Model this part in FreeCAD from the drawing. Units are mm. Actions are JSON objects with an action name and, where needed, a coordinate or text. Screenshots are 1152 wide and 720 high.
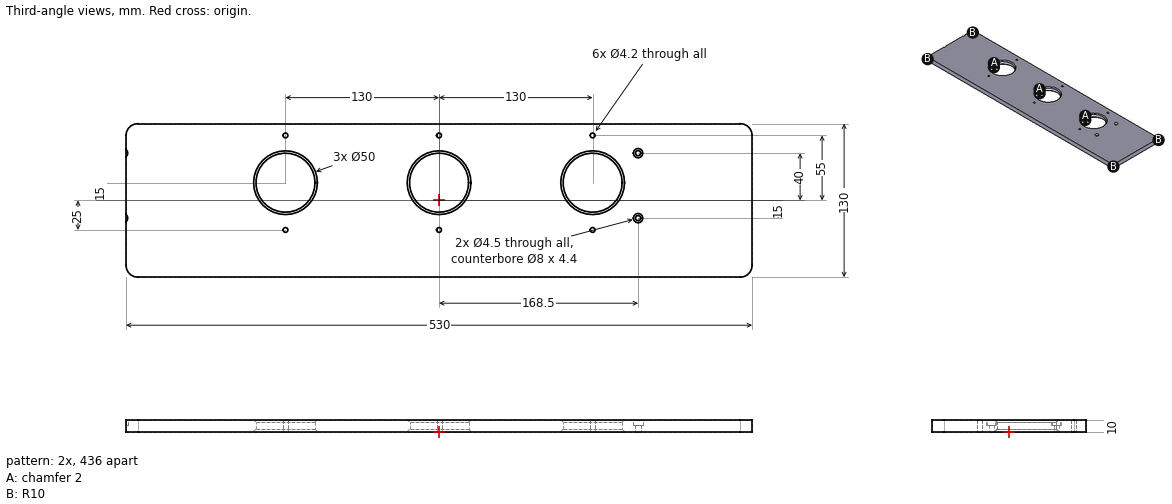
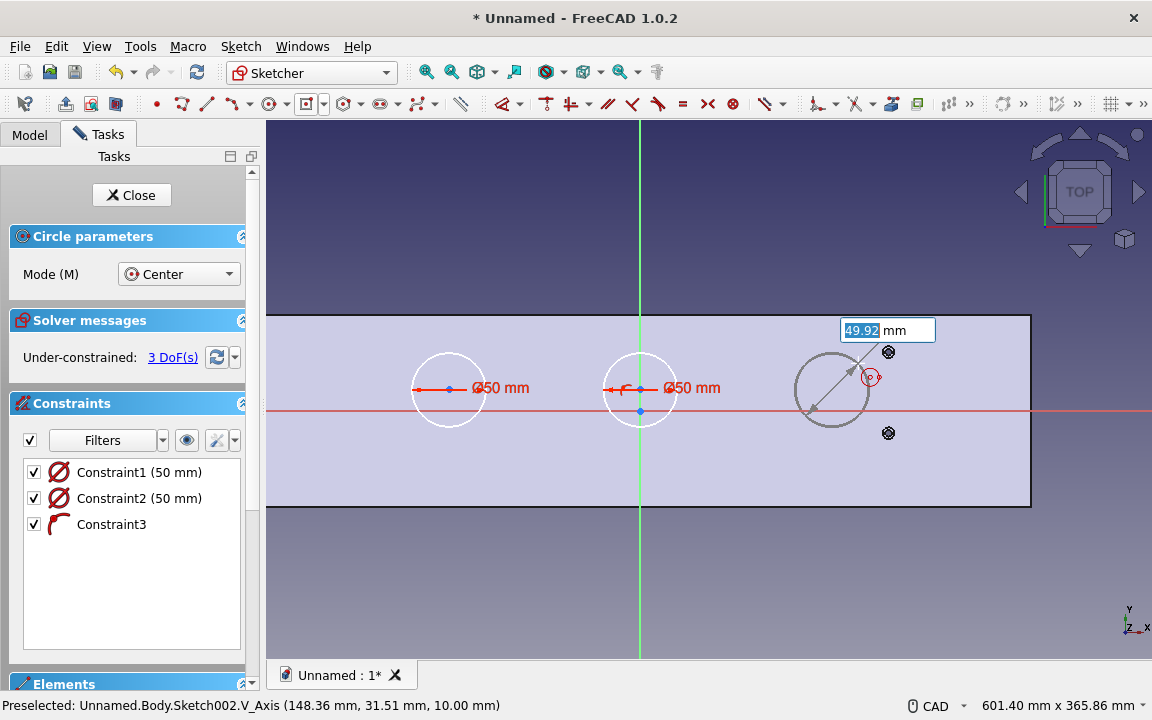
{"action": "type", "text": "50"}
{"action": "key", "text": "Return"}
{"action": "key", "text": "Escape"}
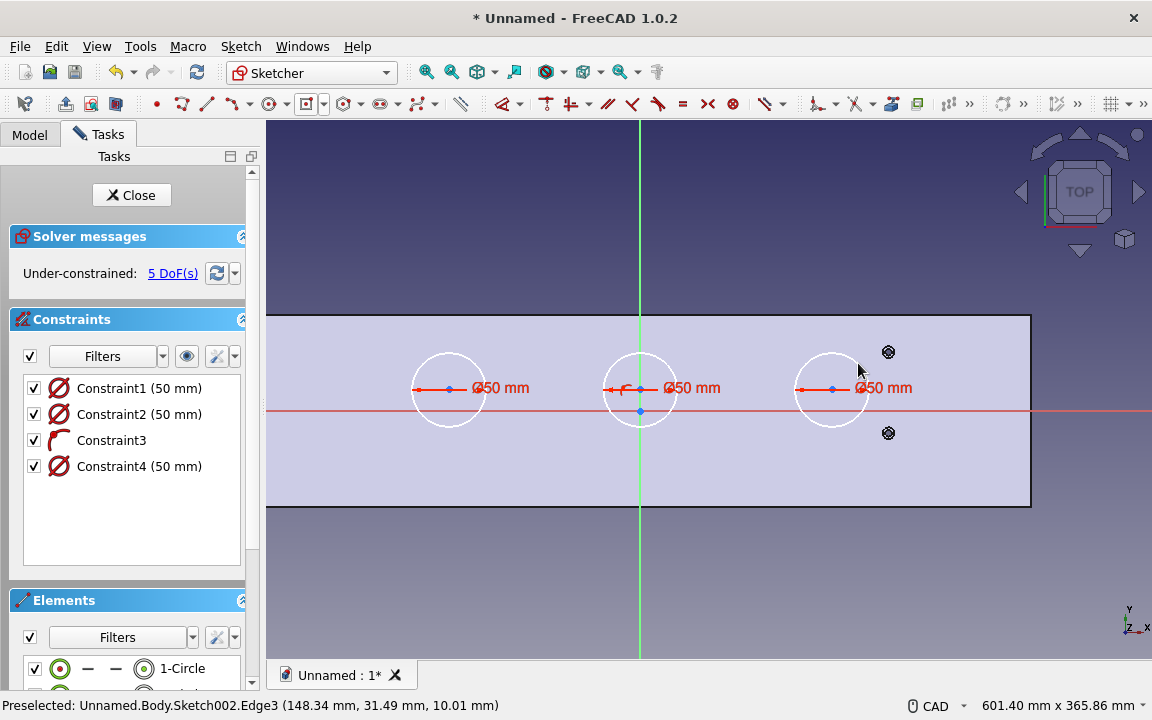
{"action": "left_click", "coordinate": [449, 390]}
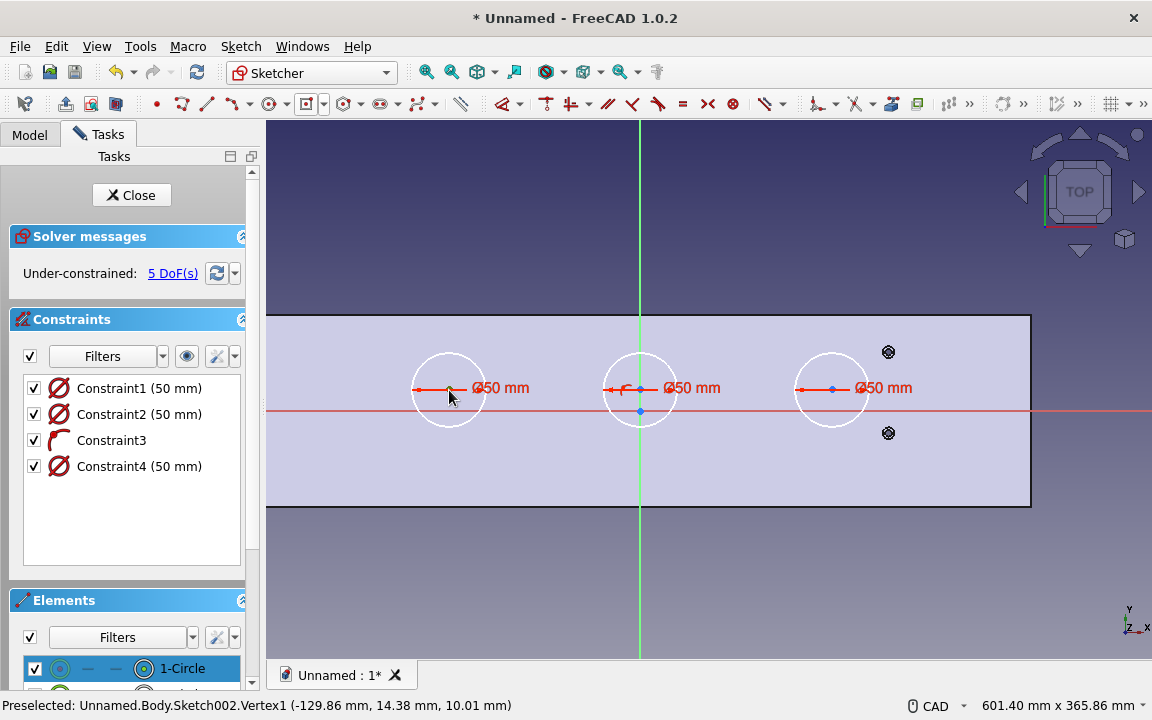
{"action": "left_click", "coordinate": [640, 390]}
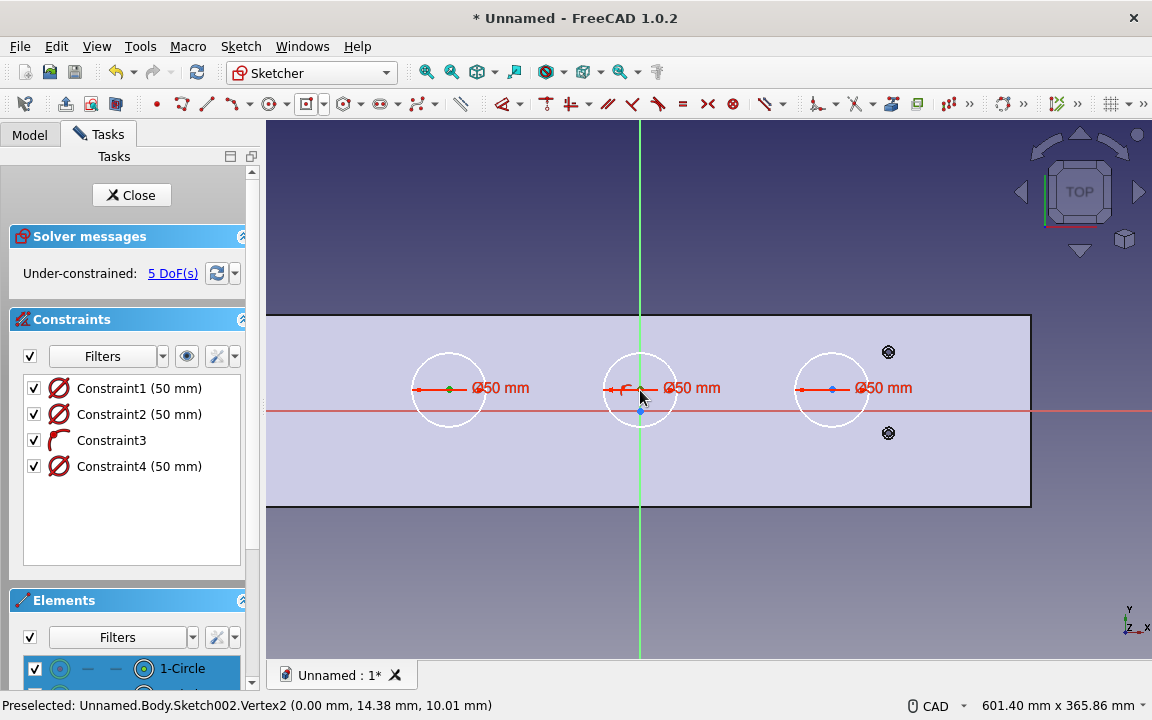
{"action": "left_click", "coordinate": [588, 104]}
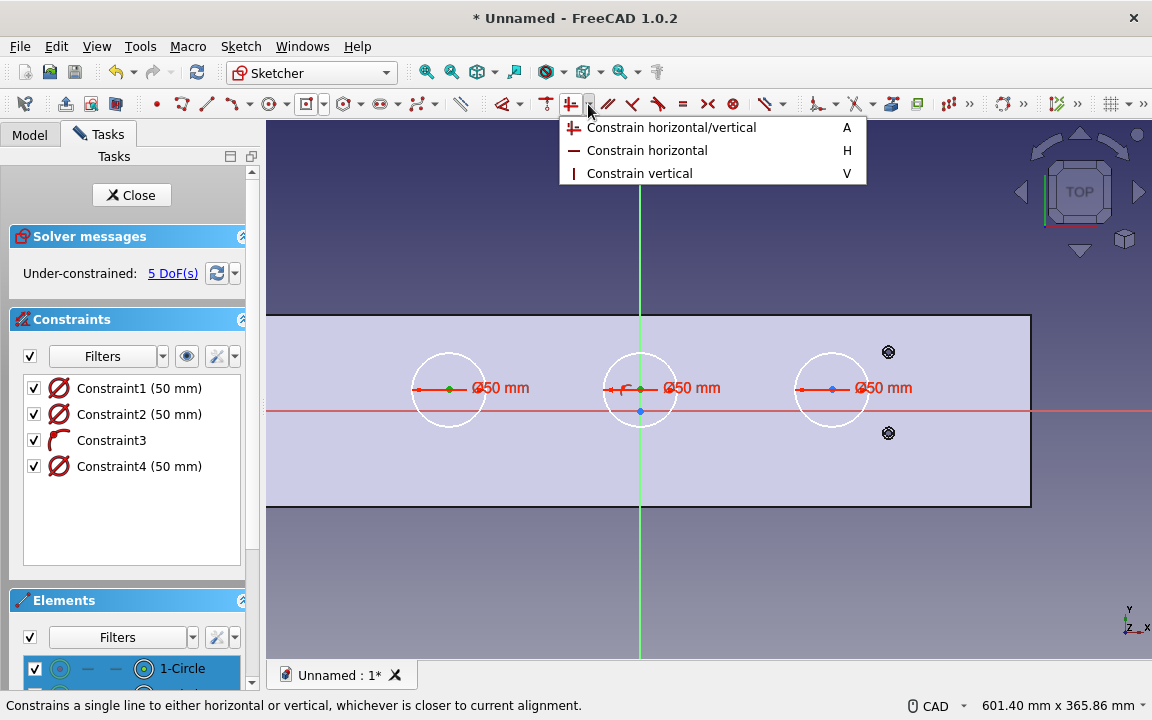
{"action": "left_click", "coordinate": [713, 150]}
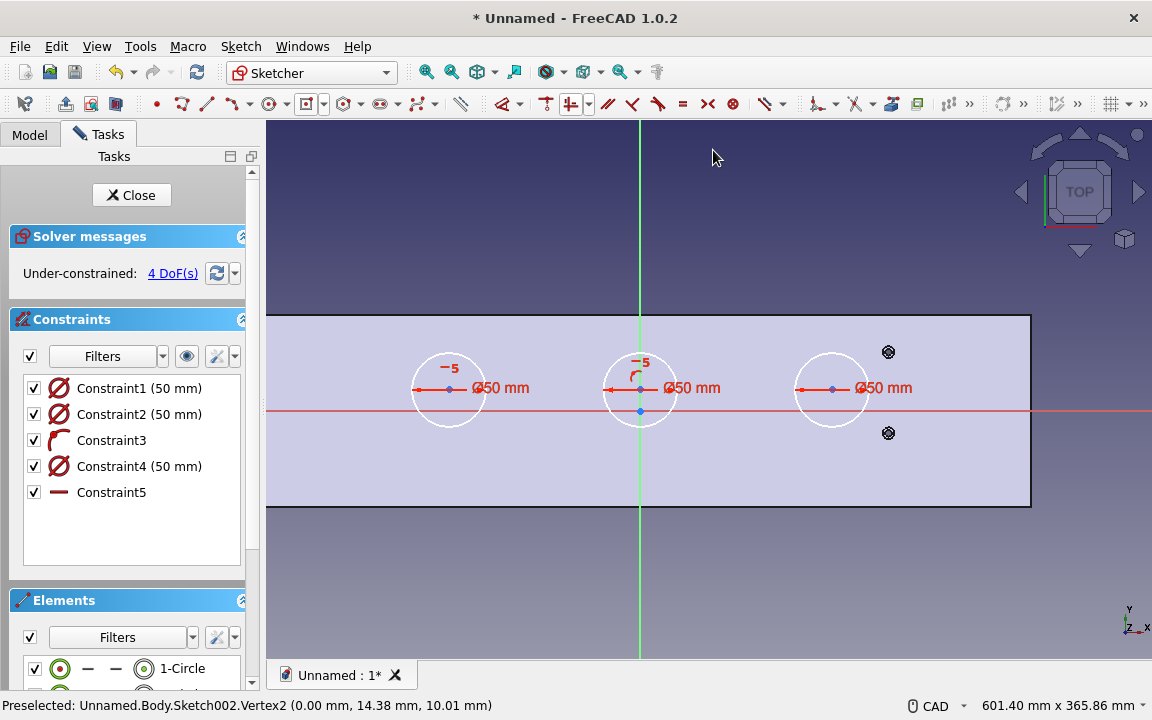
{"action": "left_click", "coordinate": [640, 390]}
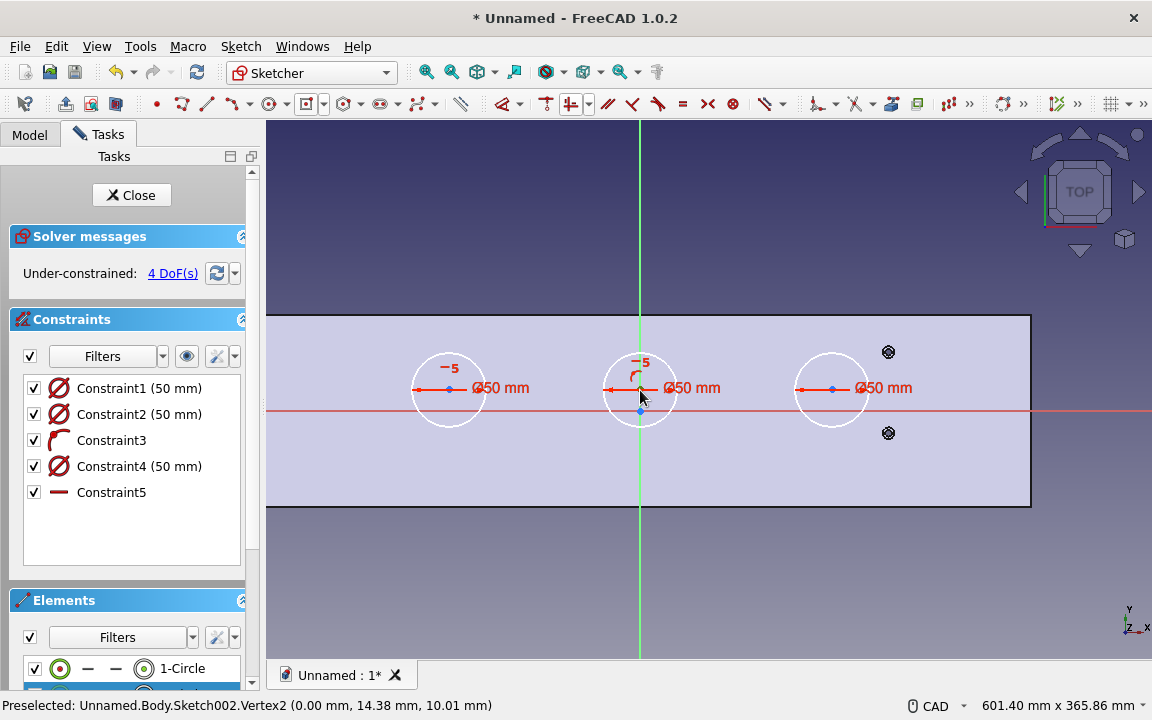
{"action": "left_click", "coordinate": [832, 390]}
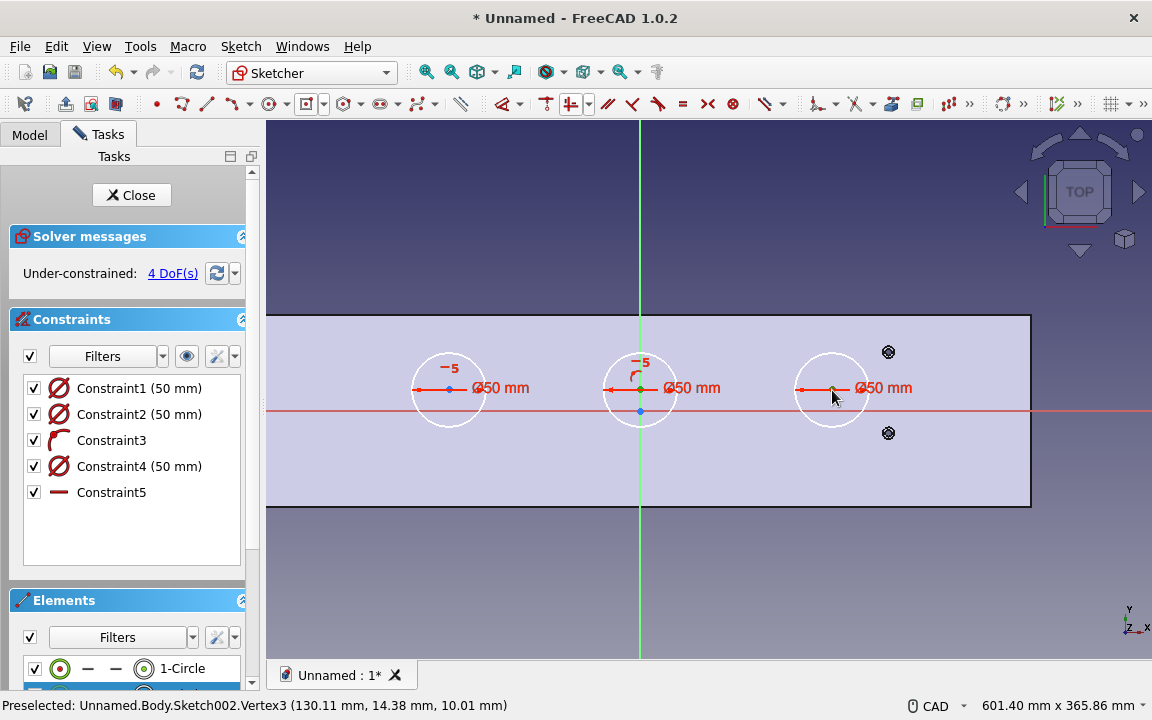
{"action": "left_click", "coordinate": [588, 104]}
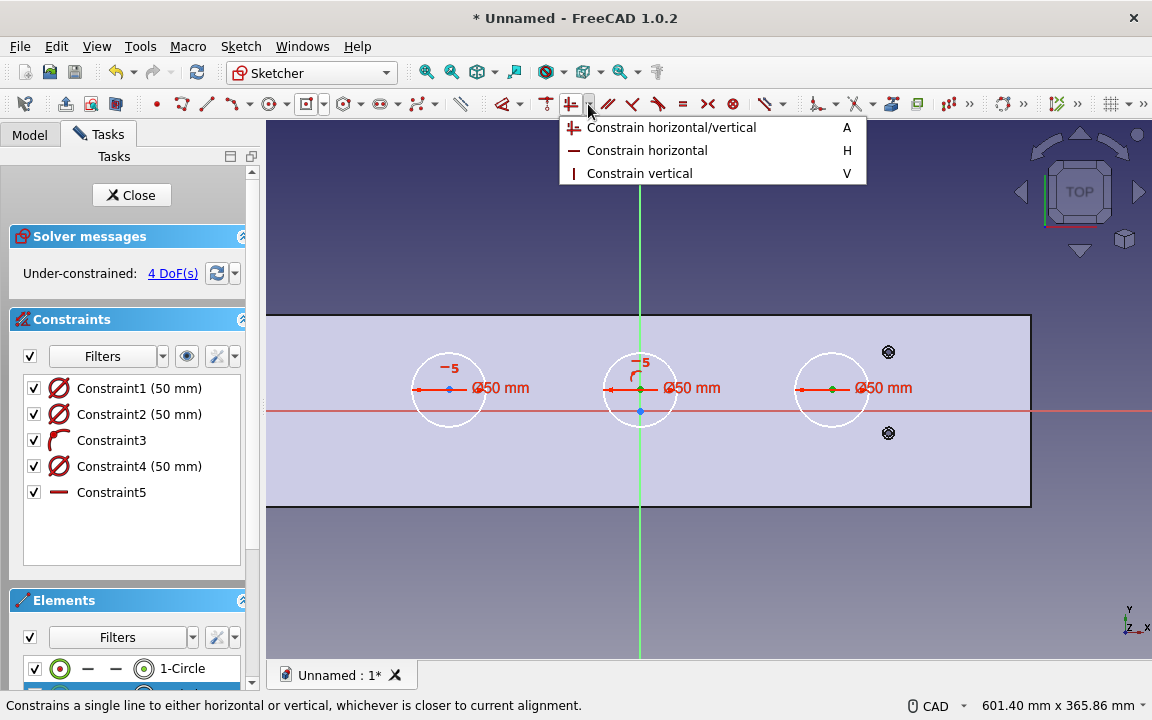
{"action": "left_click", "coordinate": [713, 150]}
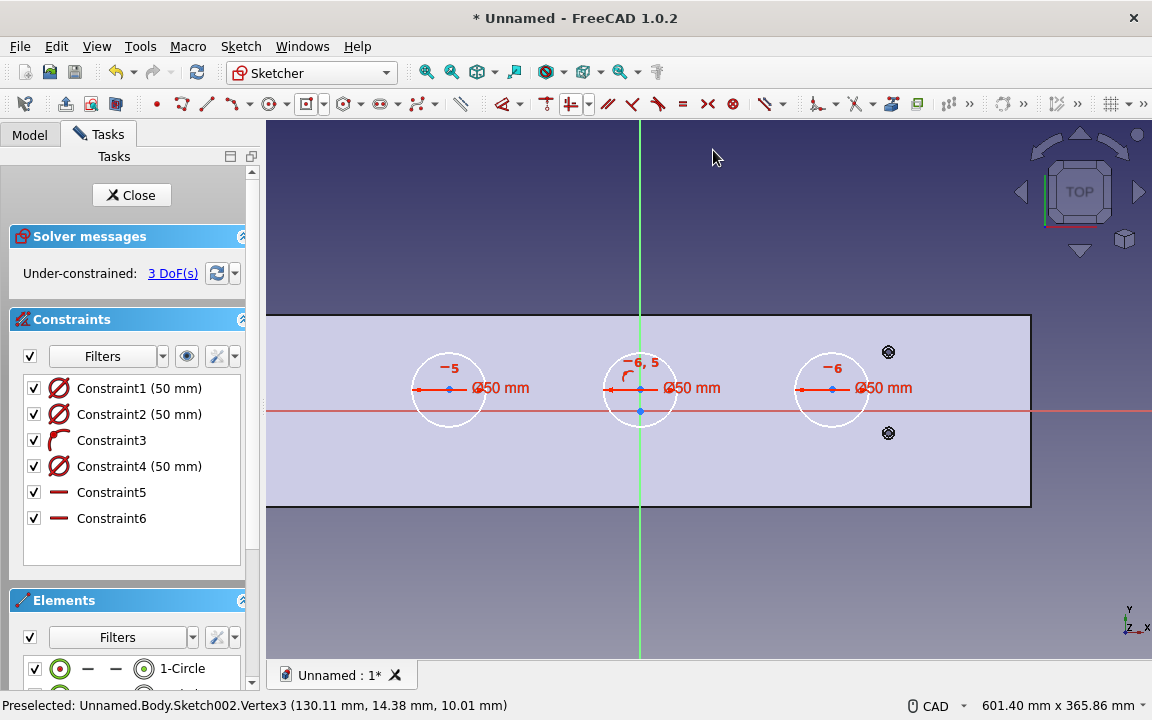
{"action": "left_click", "coordinate": [502, 104]}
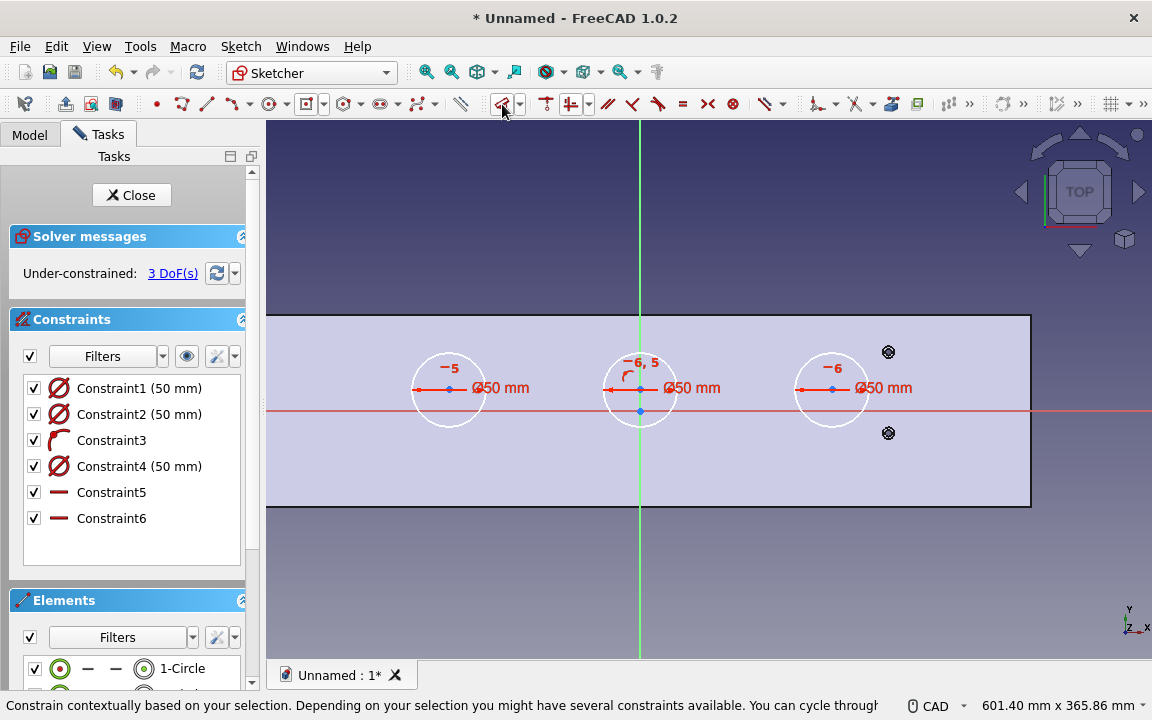
{"action": "scroll", "coordinate": [449, 390], "scroll_direction": "up", "scroll_amount": 3}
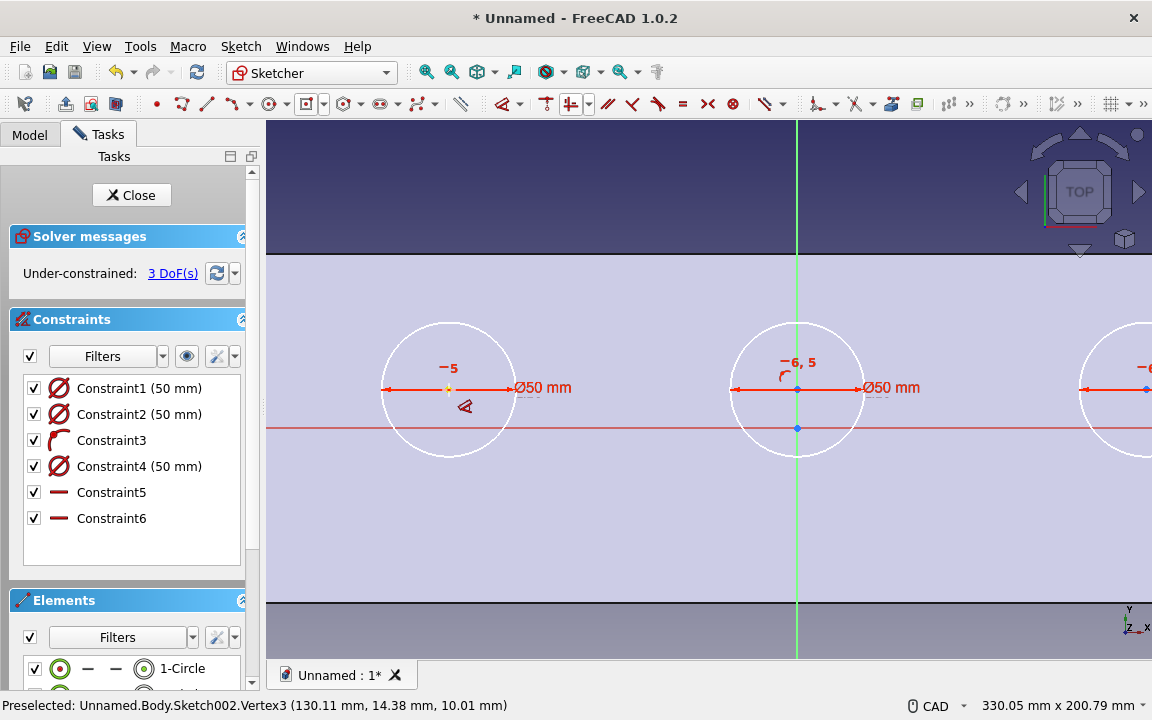
{"action": "left_click", "coordinate": [449, 390]}
{"action": "left_click", "coordinate": [415, 409]}